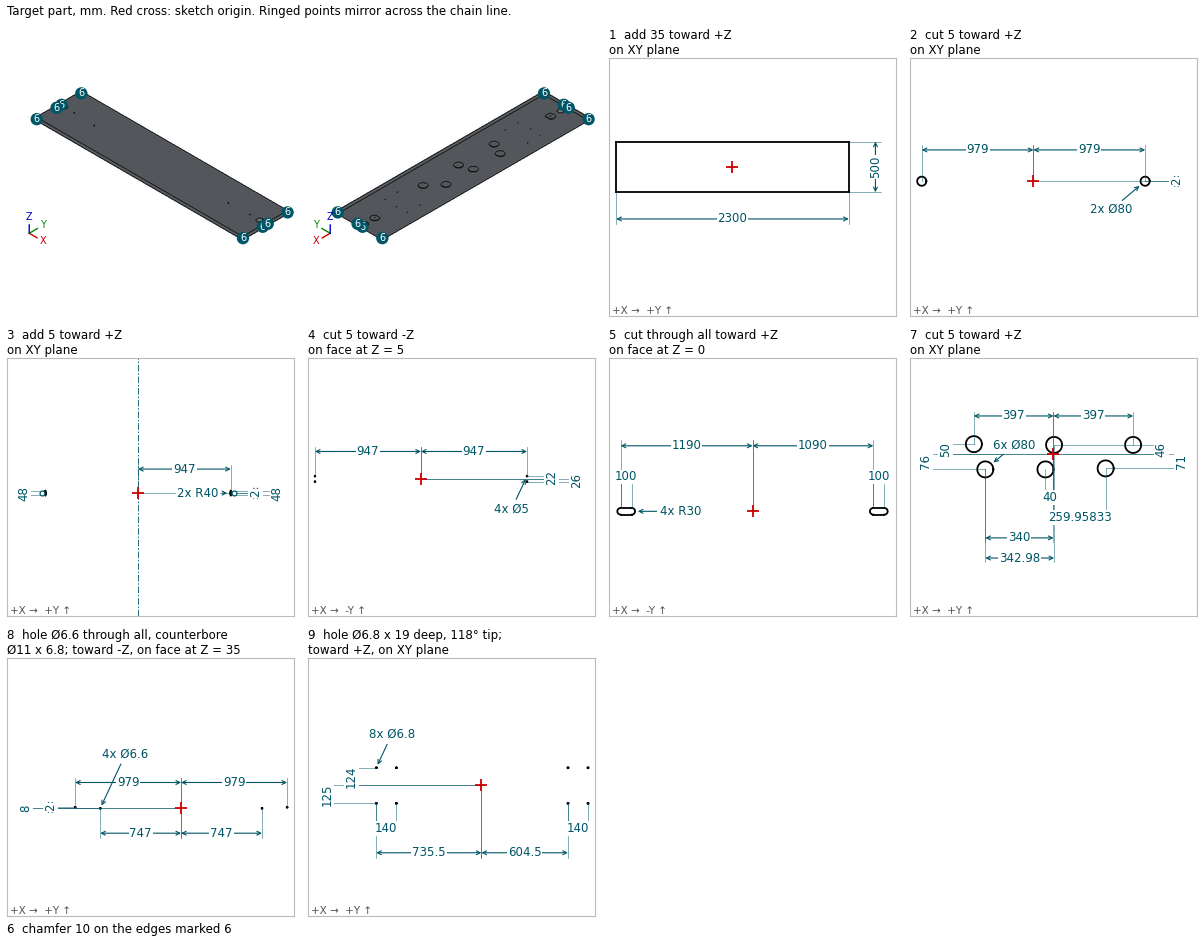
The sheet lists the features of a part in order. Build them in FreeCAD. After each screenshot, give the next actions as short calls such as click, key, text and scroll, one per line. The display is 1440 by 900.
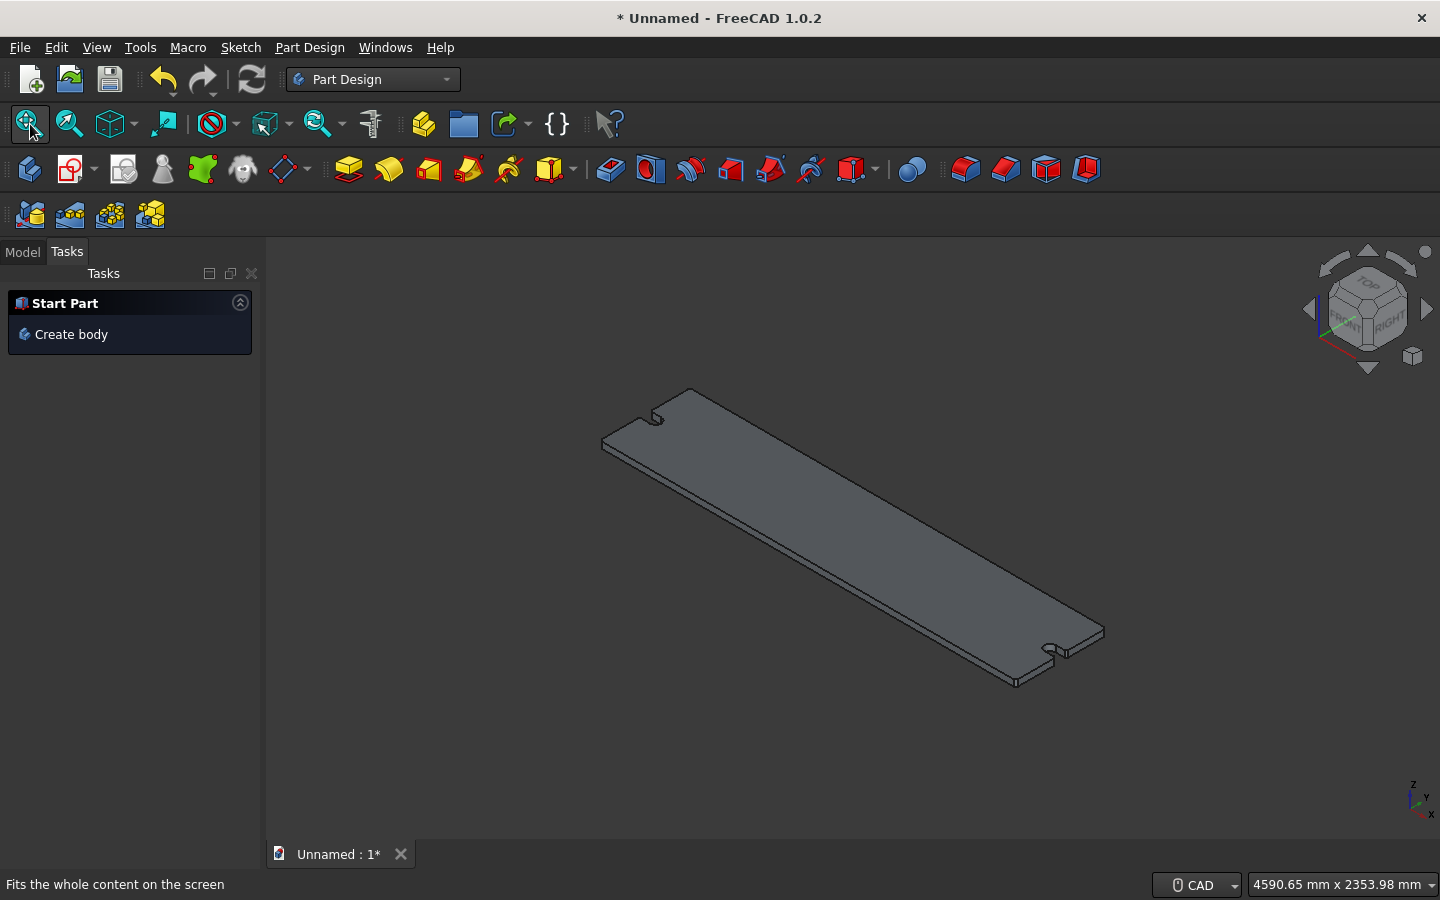
click(972, 602)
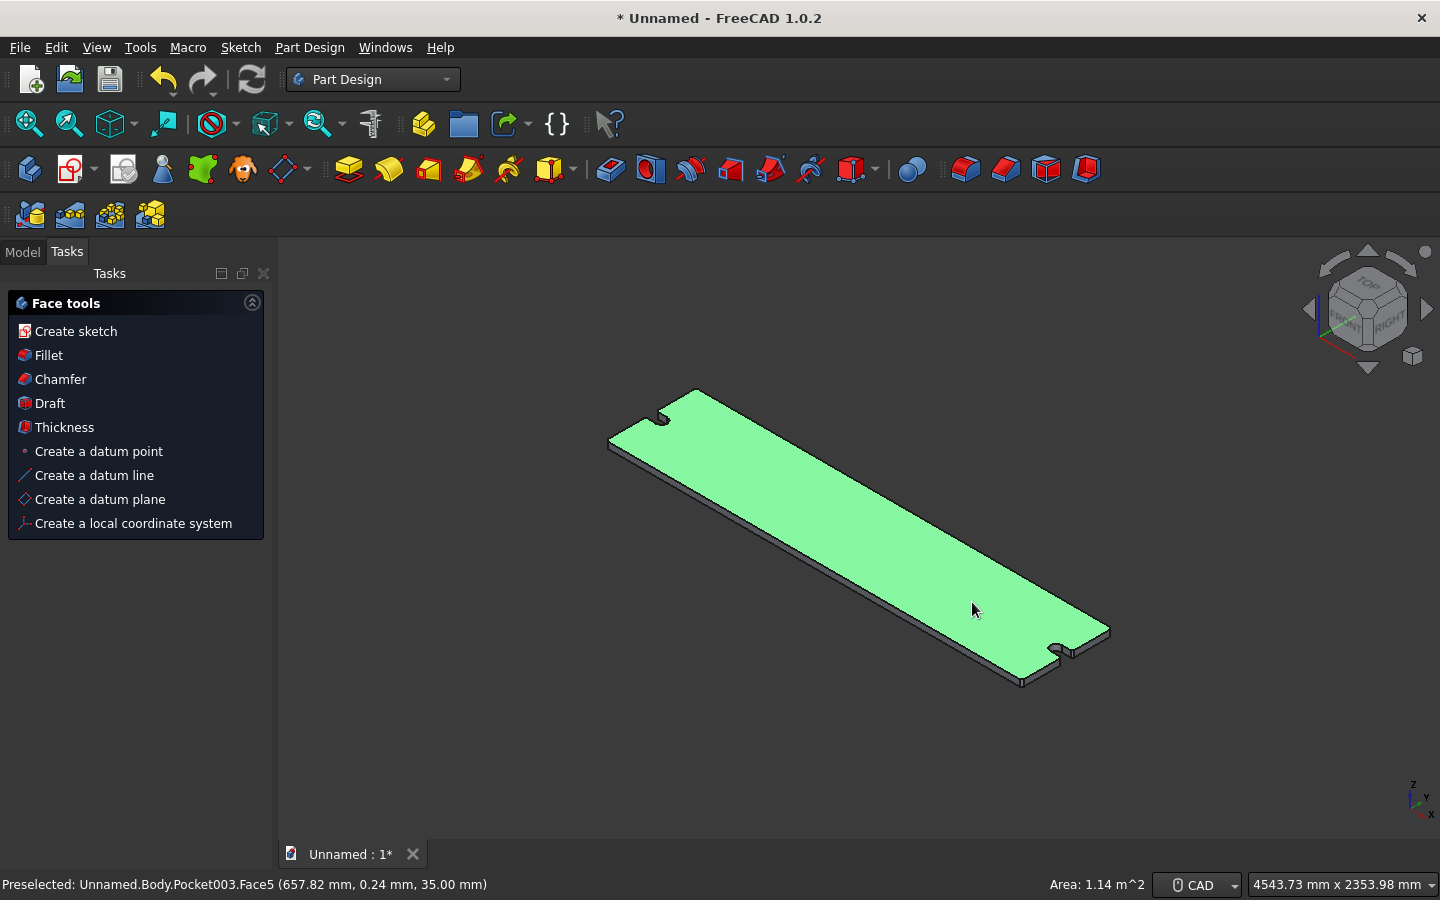
click(70, 170)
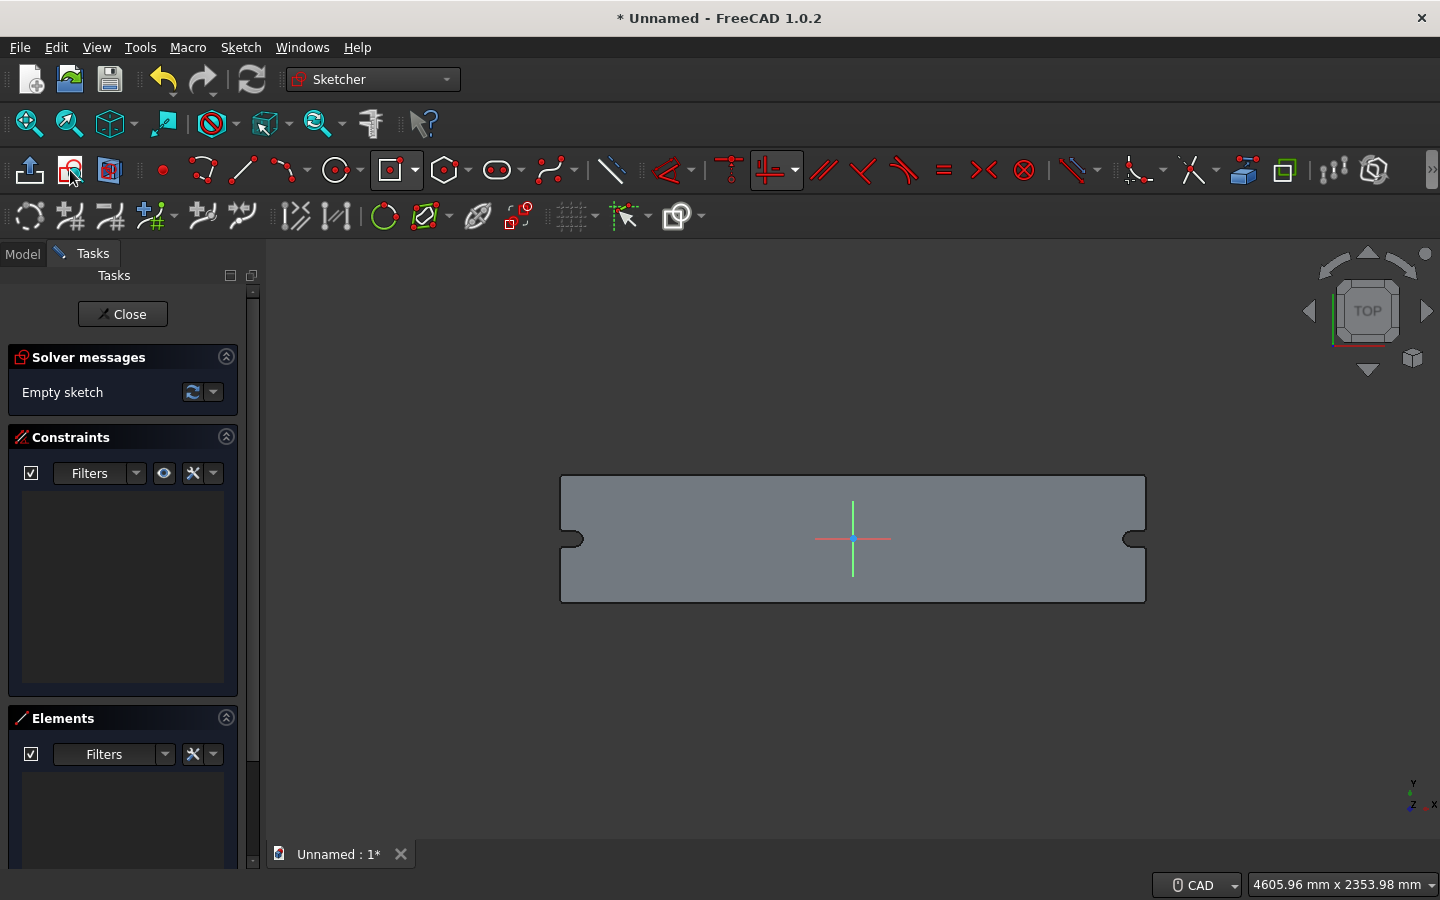
scroll(992, 541, up, 2)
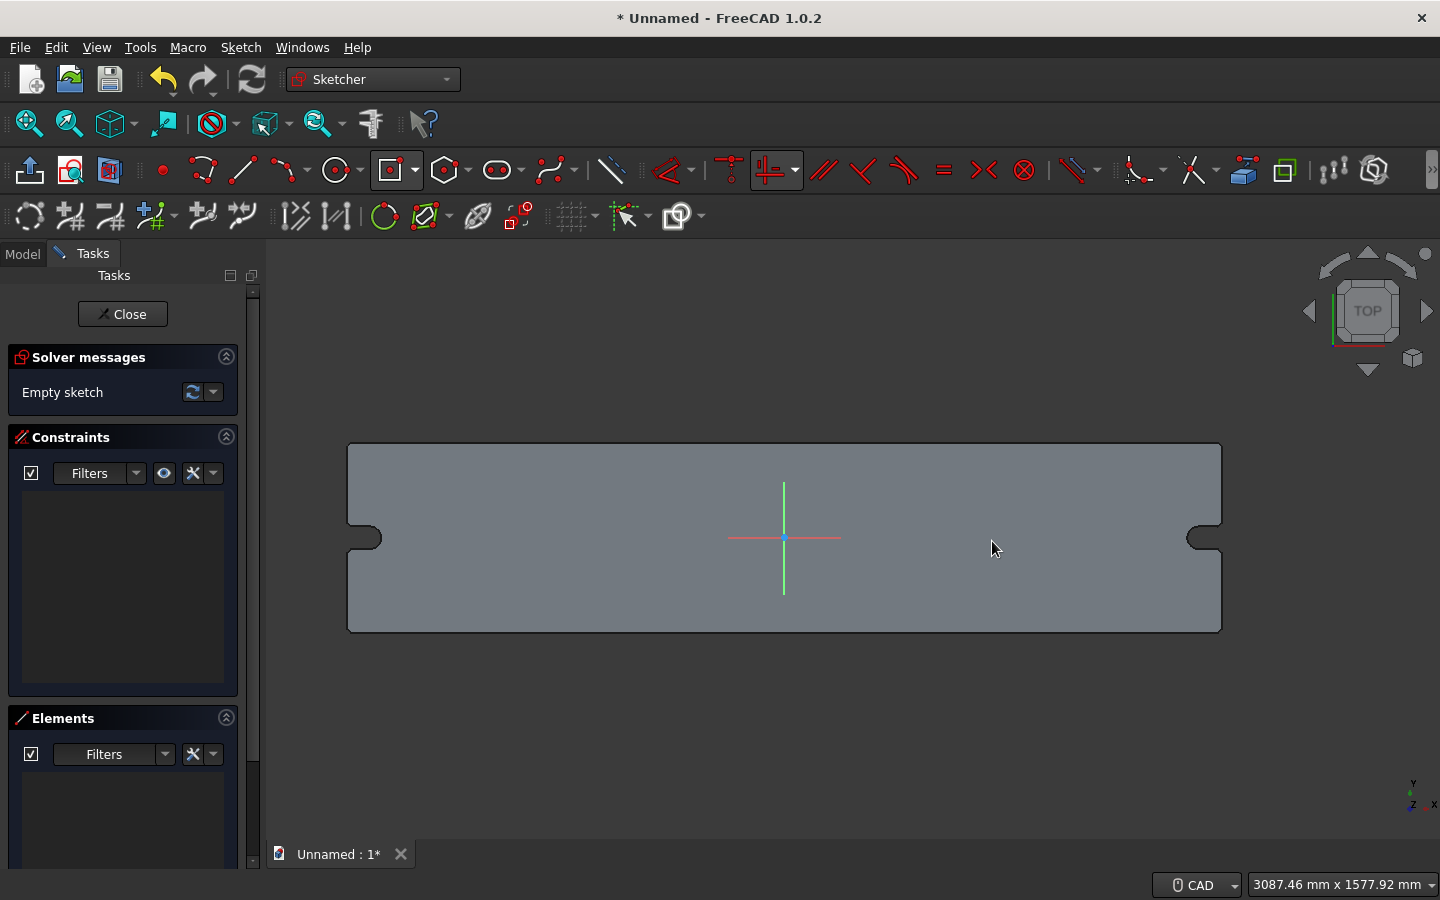
click(336, 170)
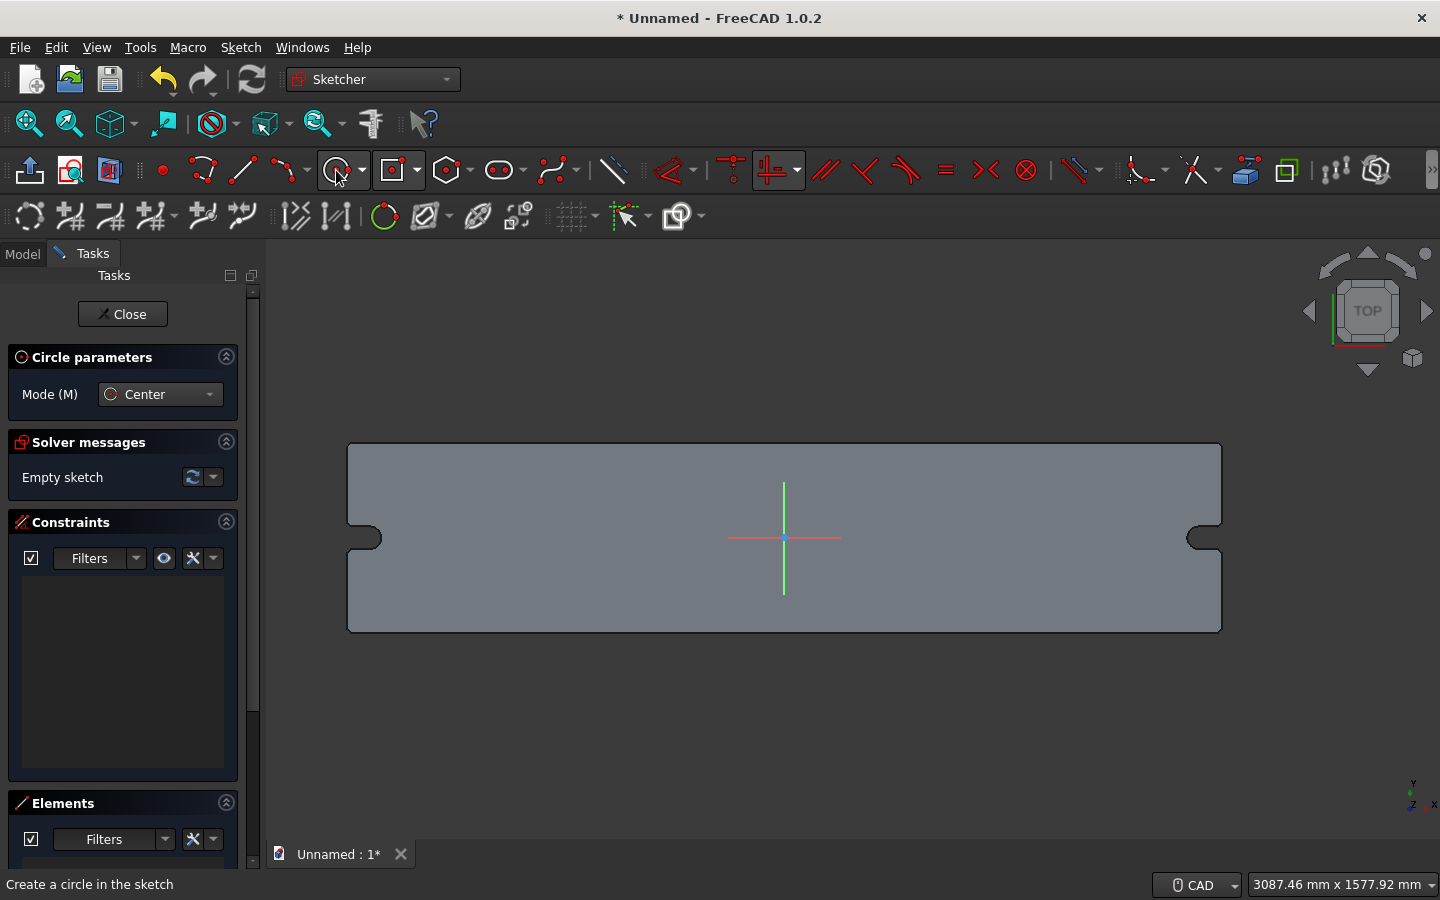
scroll(500, 541, up, 15)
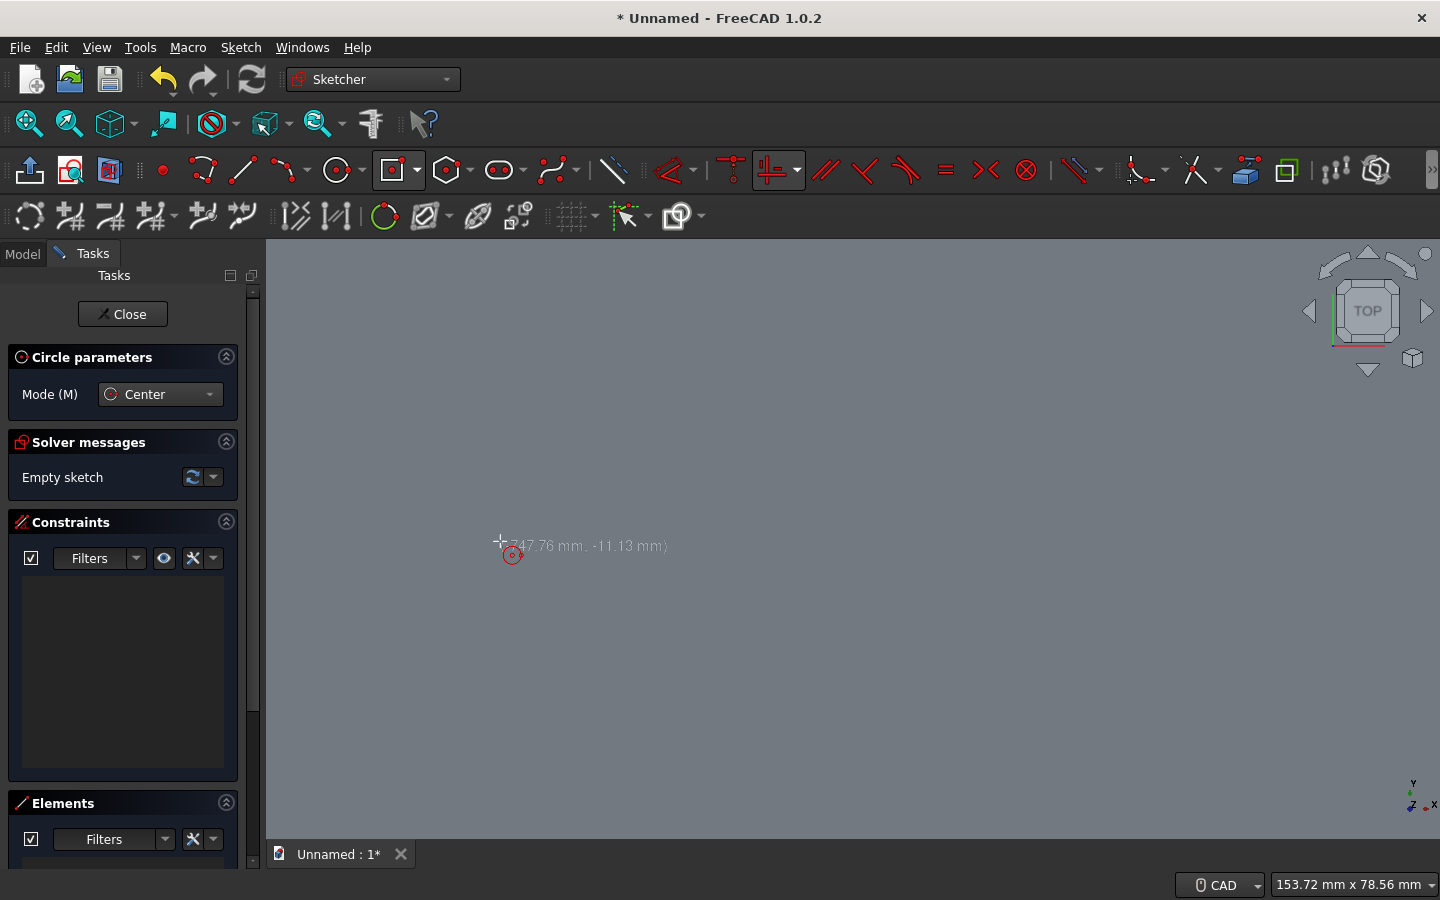
scroll(500, 542, down, 15)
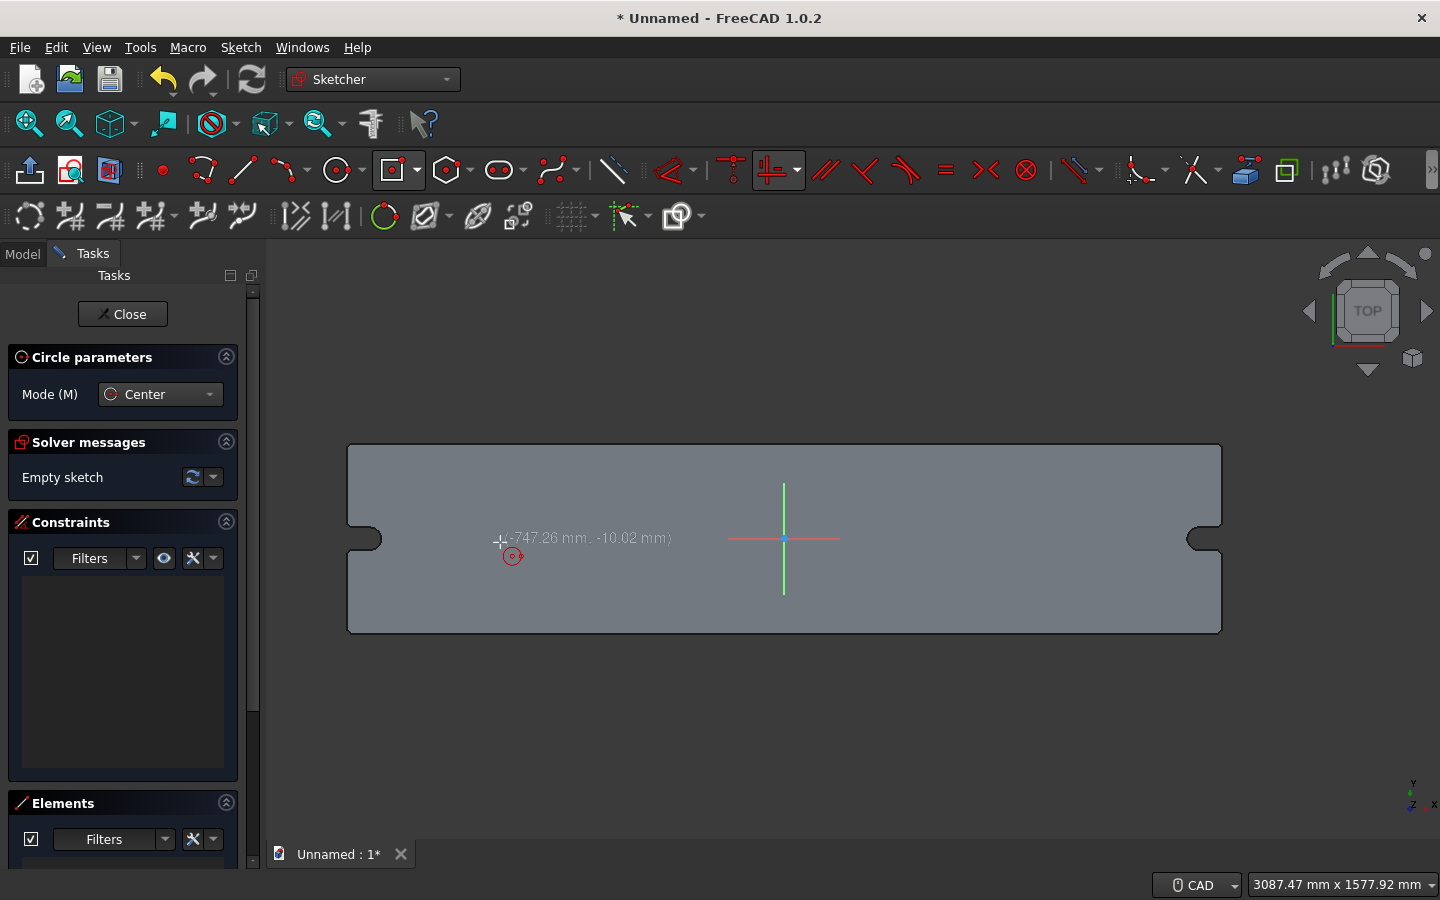
scroll(500, 542, up, 9)